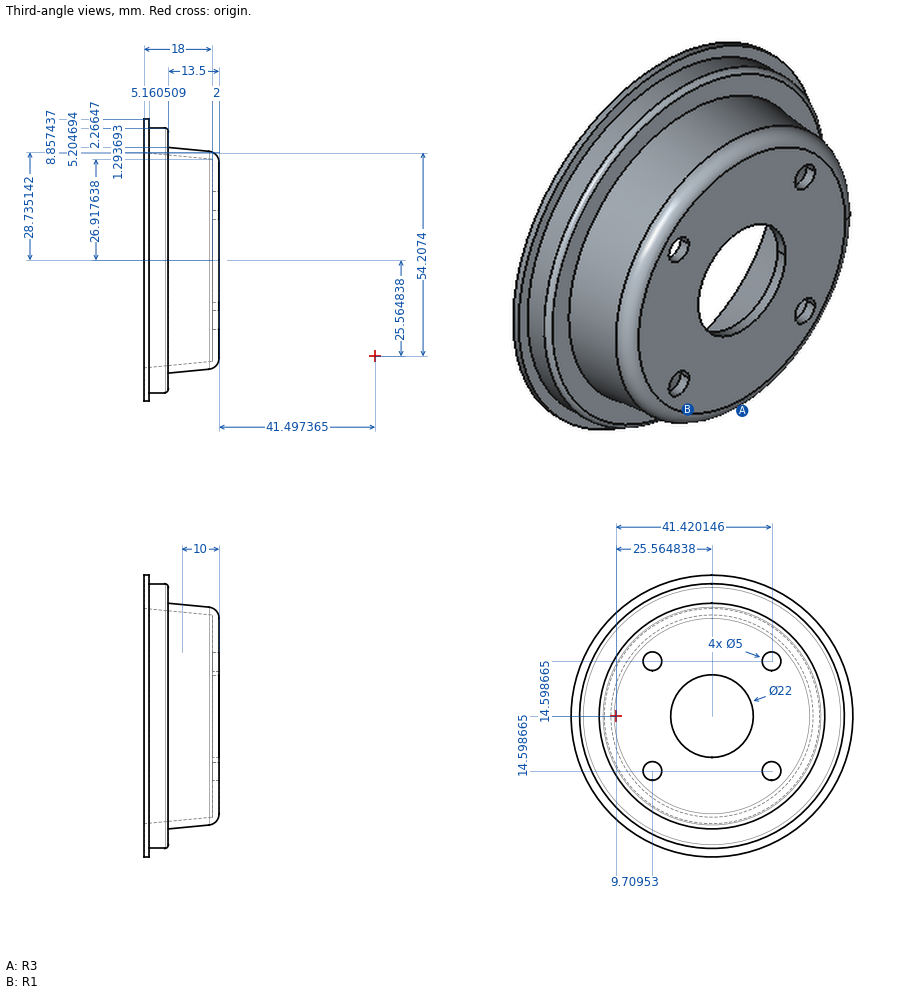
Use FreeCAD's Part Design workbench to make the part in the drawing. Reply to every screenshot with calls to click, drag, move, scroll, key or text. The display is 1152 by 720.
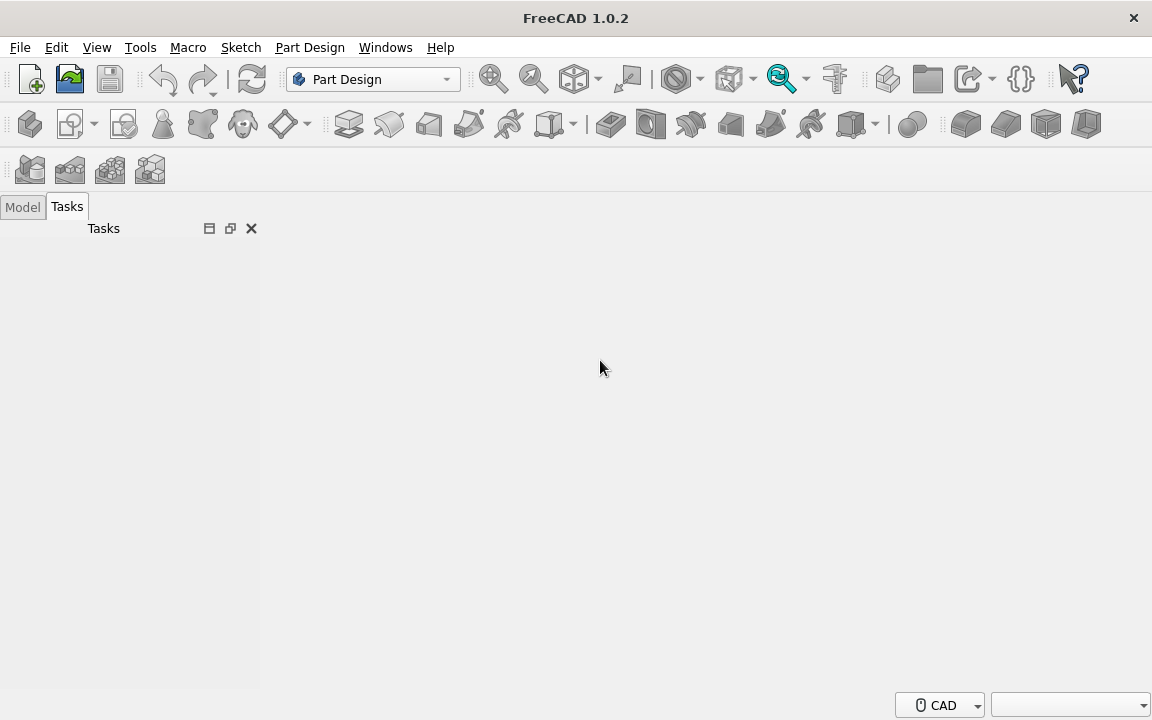
key(ctrl+n)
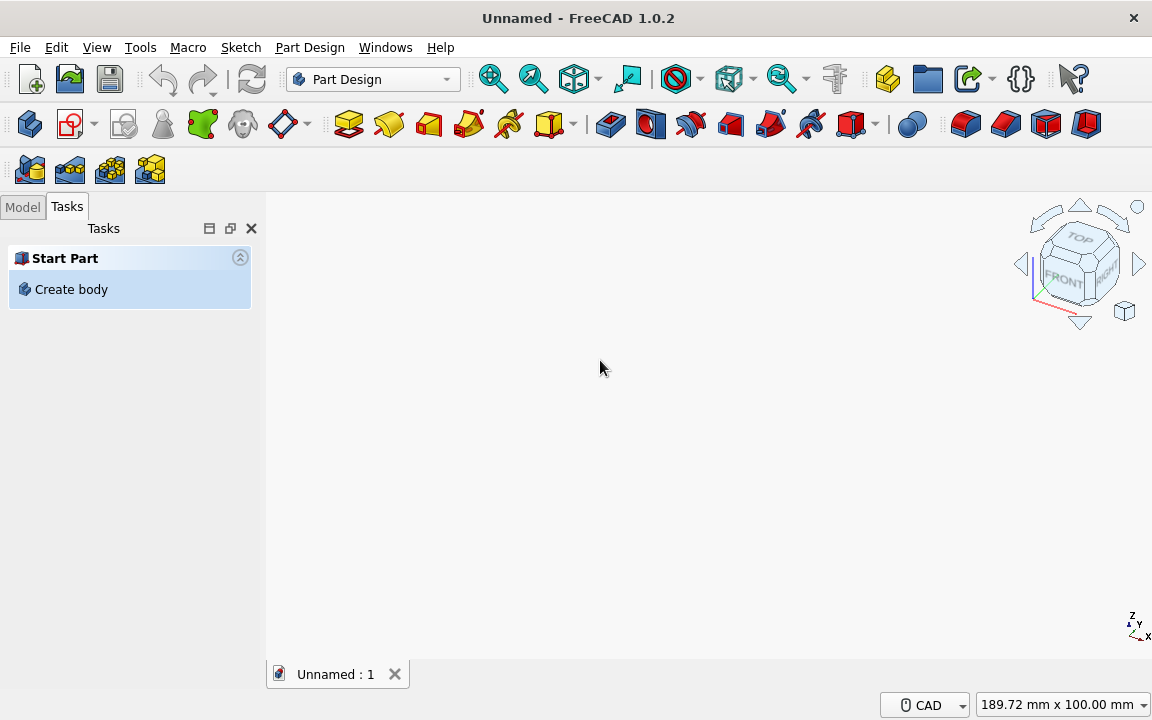
click(70, 124)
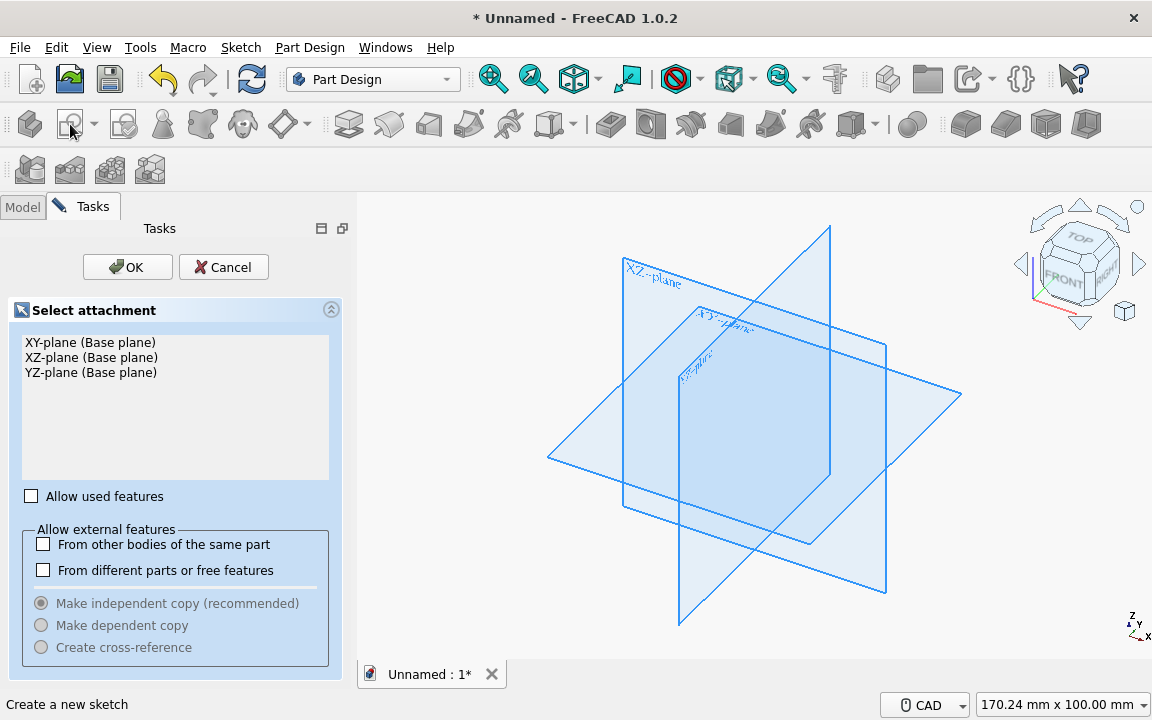
click(82, 342)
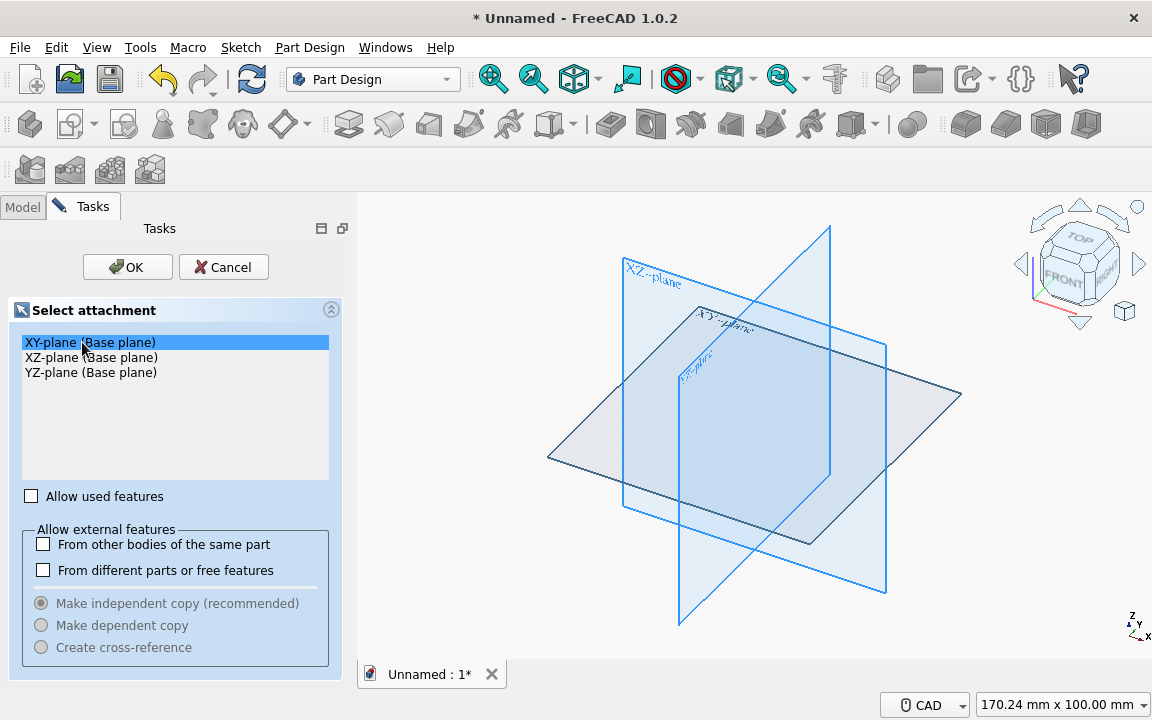
click(128, 267)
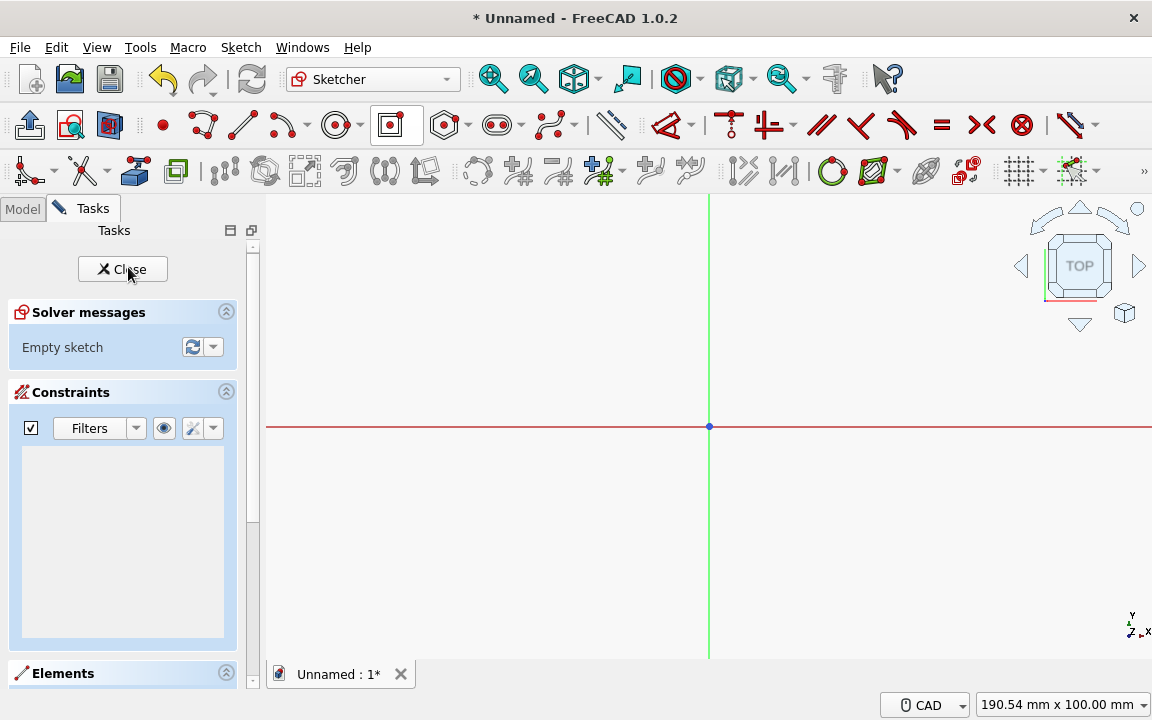
scroll(792, 631, down, 2)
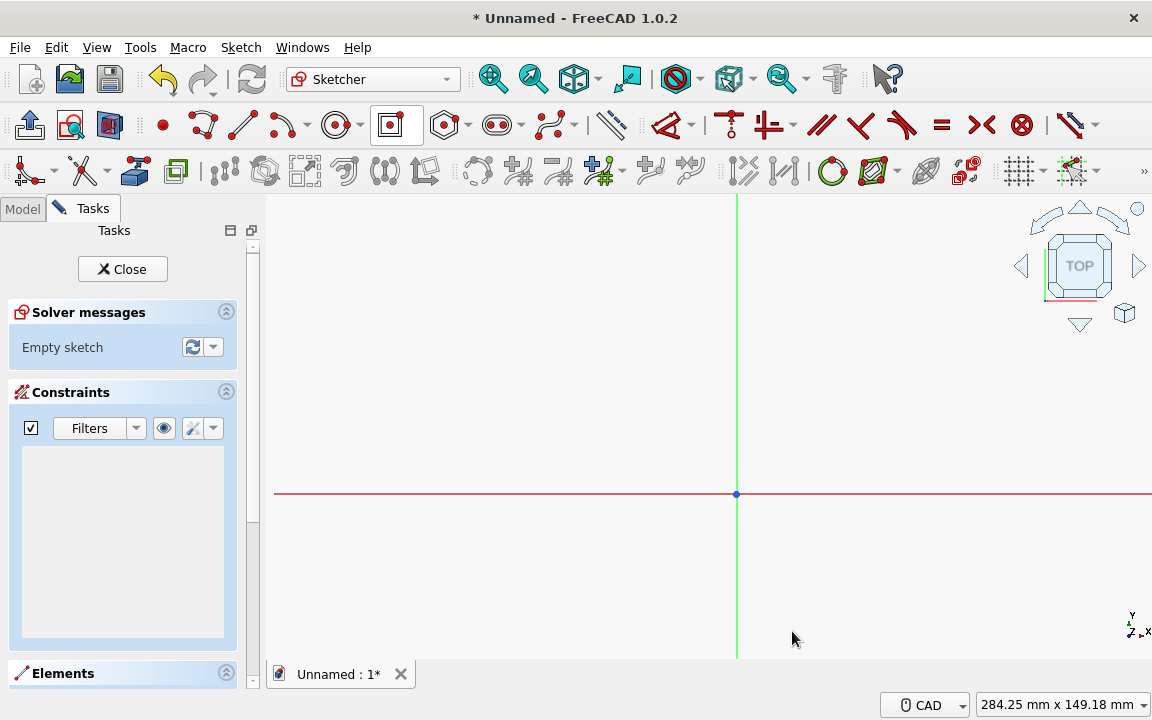
scroll(641, 334, up, 2)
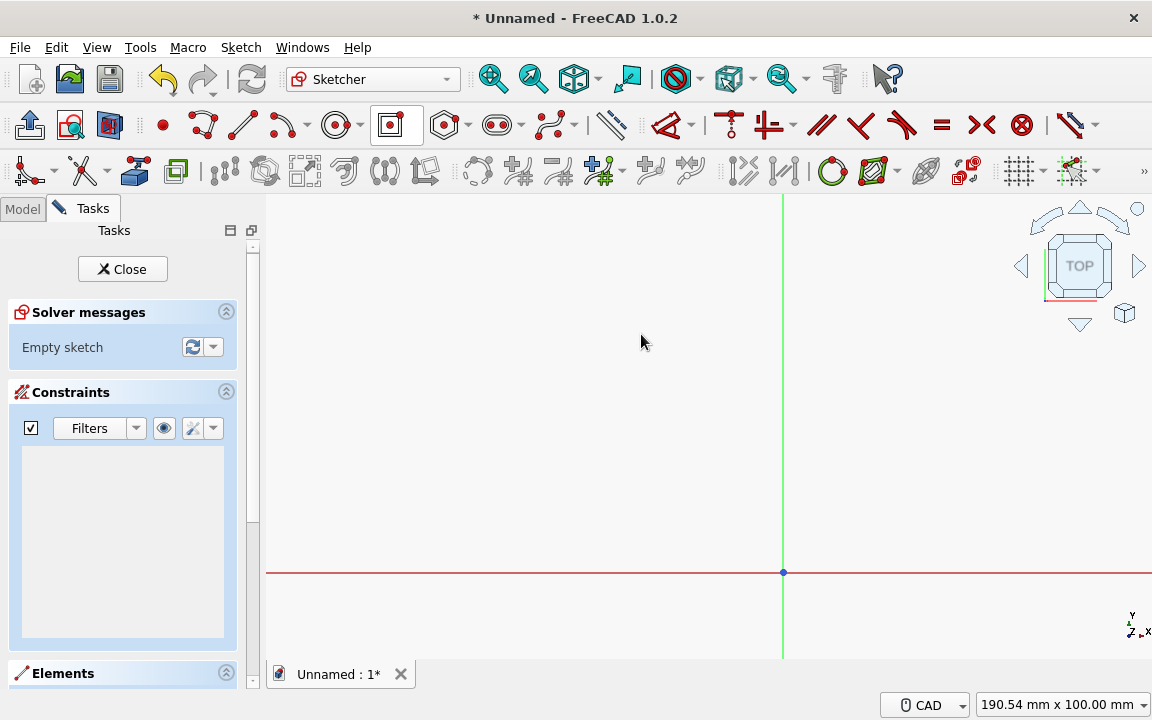
key(g)
key(m)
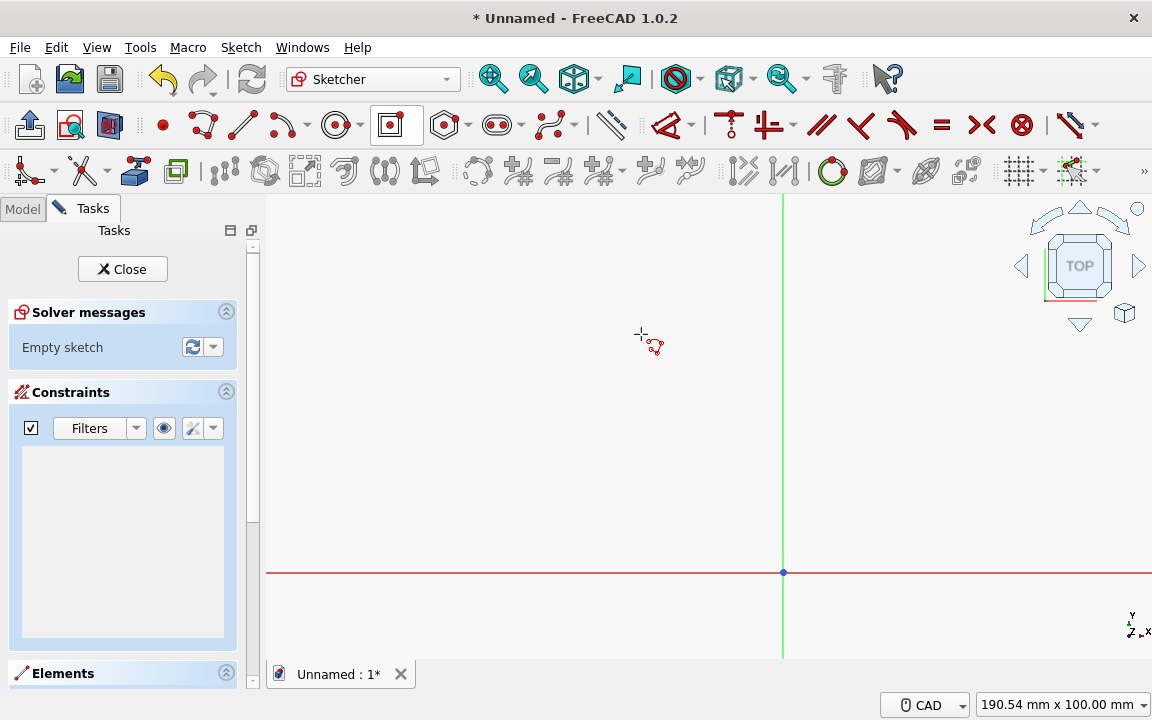
click(590, 454)
click(590, 320)
click(528, 314)
click(528, 290)
click(504, 290)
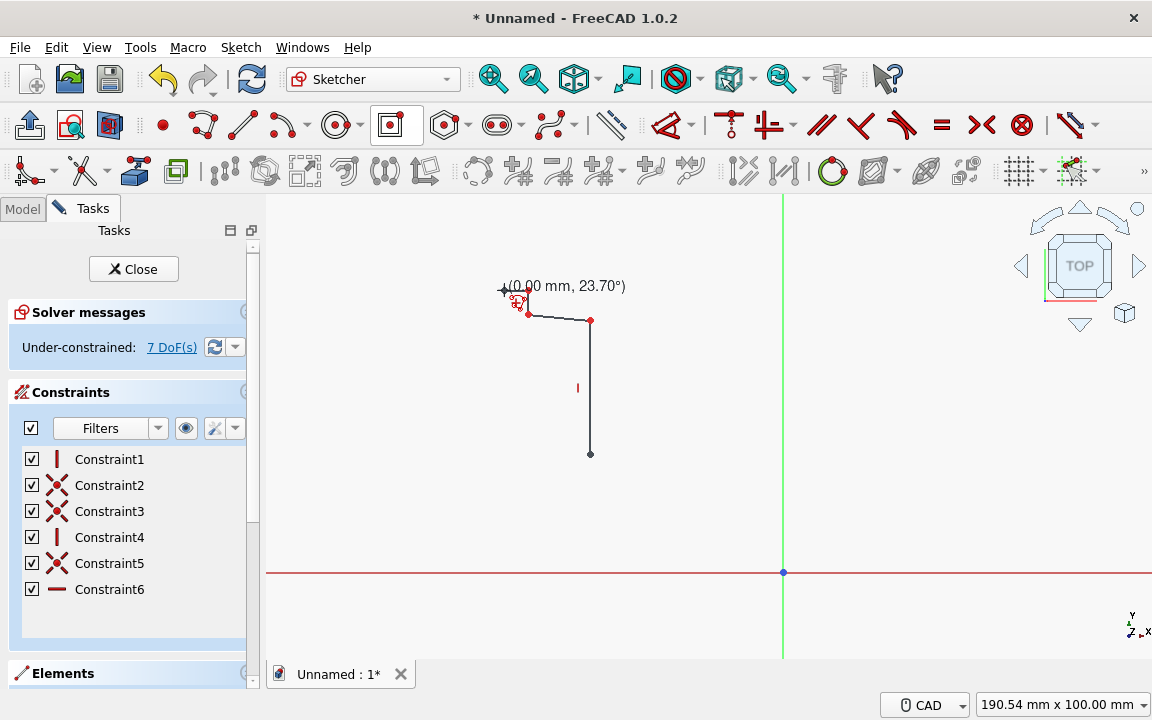
scroll(504, 280, up, 3)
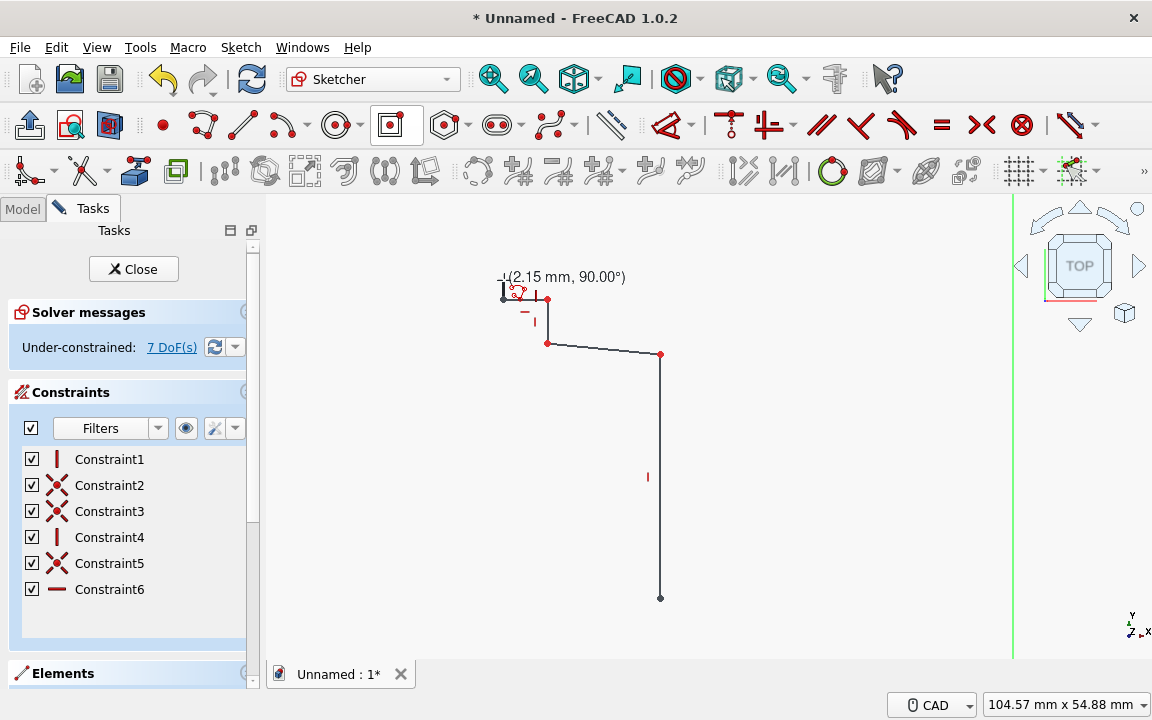
click(504, 279)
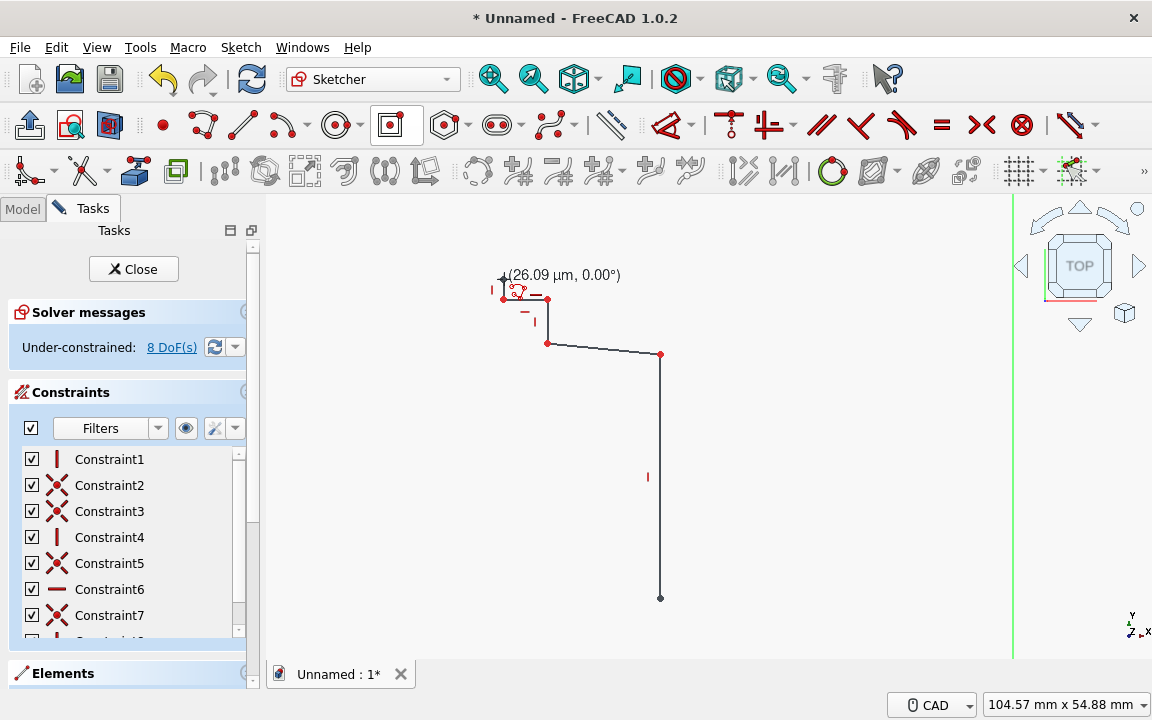
scroll(492, 279, up, 2)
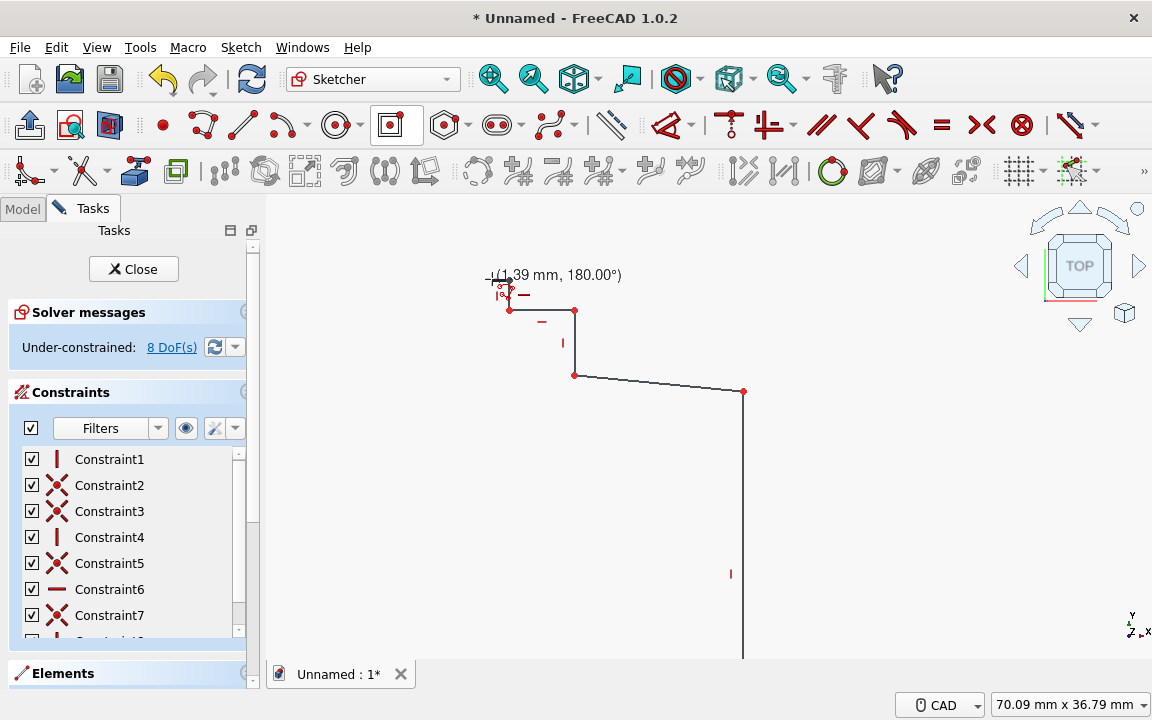
click(491, 279)
click(491, 391)
click(719, 413)